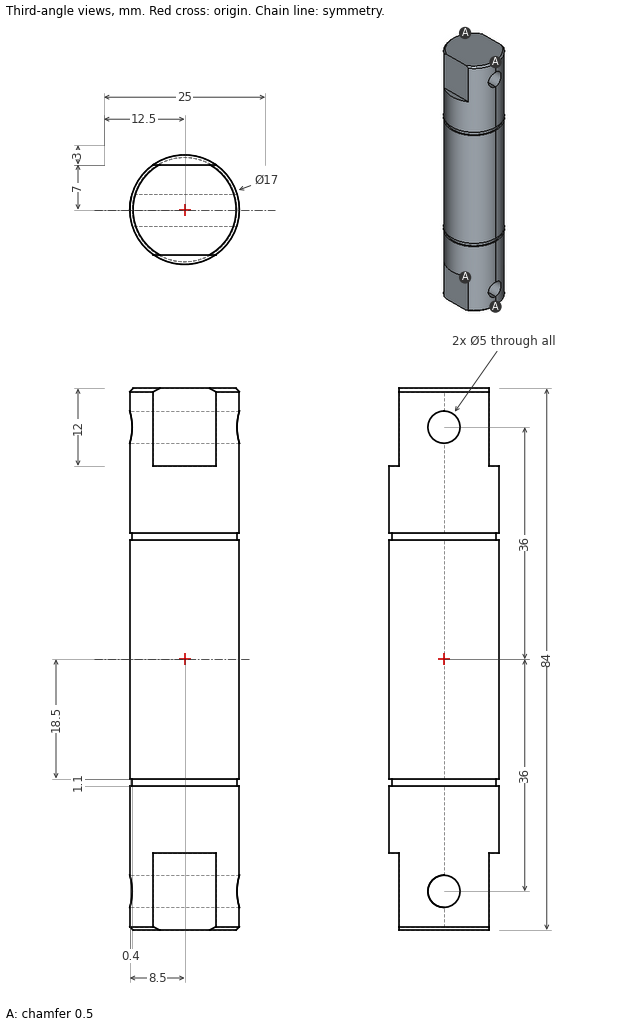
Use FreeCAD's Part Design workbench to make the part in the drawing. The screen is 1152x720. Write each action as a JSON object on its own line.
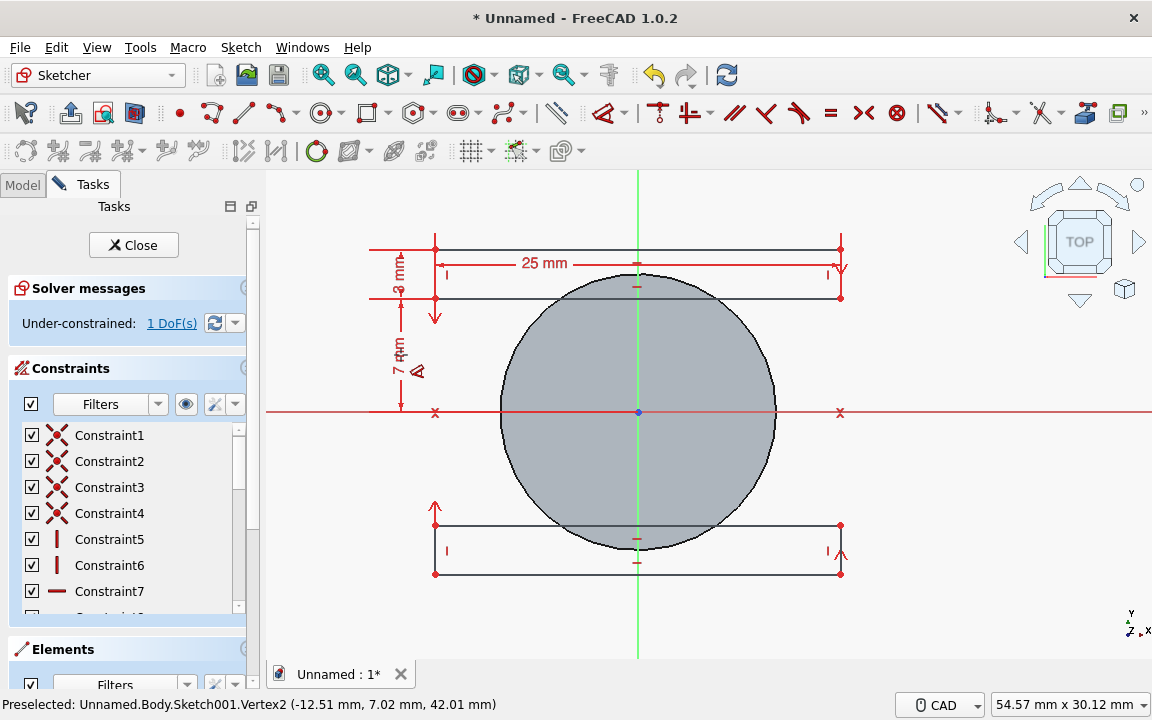
{"action": "left_click", "coordinate": [435, 250]}
{"action": "left_click", "coordinate": [537, 216]}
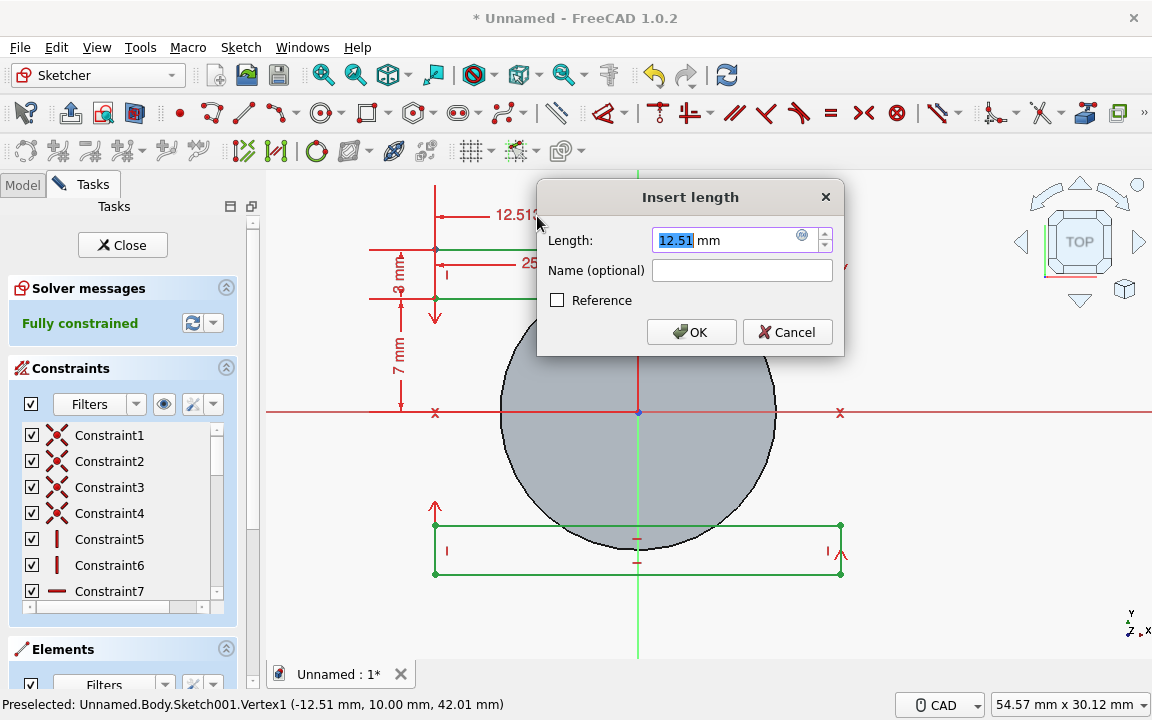
{"action": "type", "text": "12.5"}
{"action": "key", "text": "Return"}
{"action": "key", "text": "Escape"}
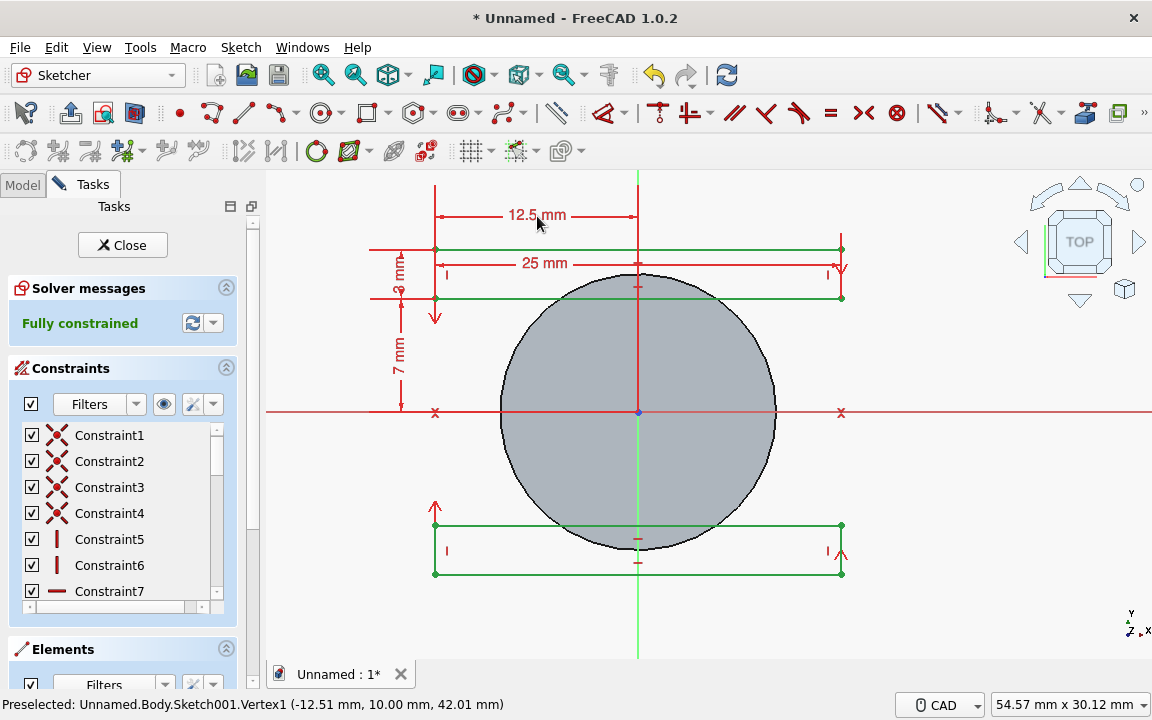
{"action": "left_click", "coordinate": [123, 245]}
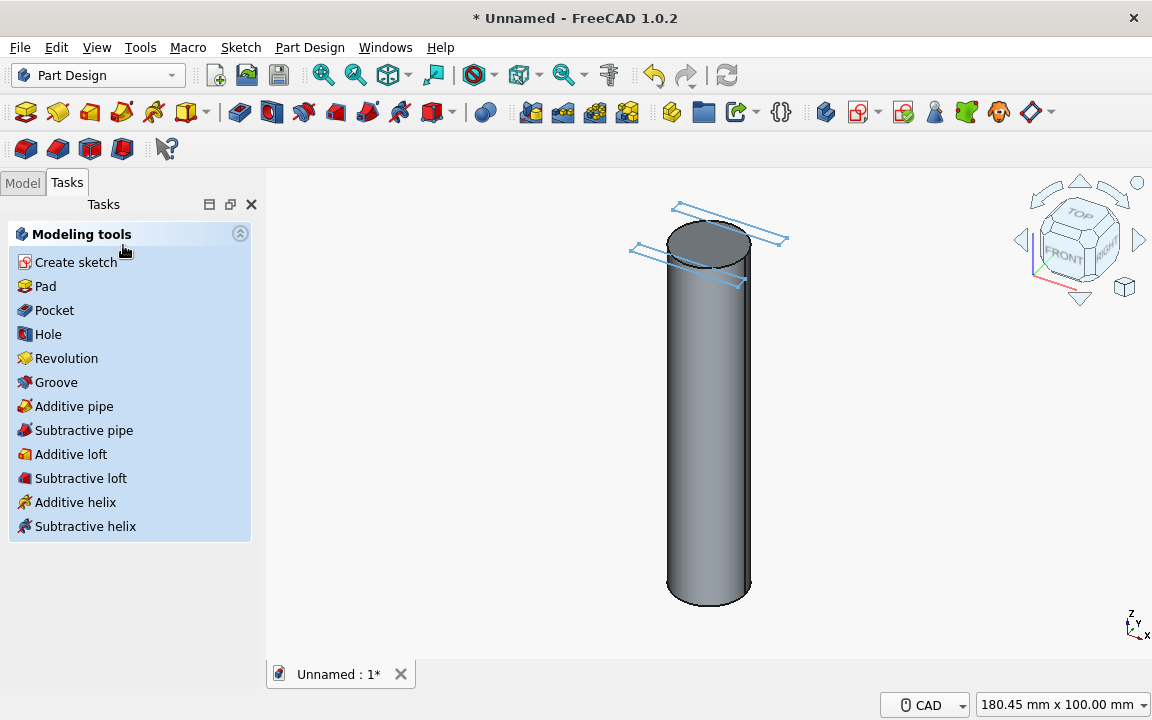
{"action": "left_click", "coordinate": [240, 112]}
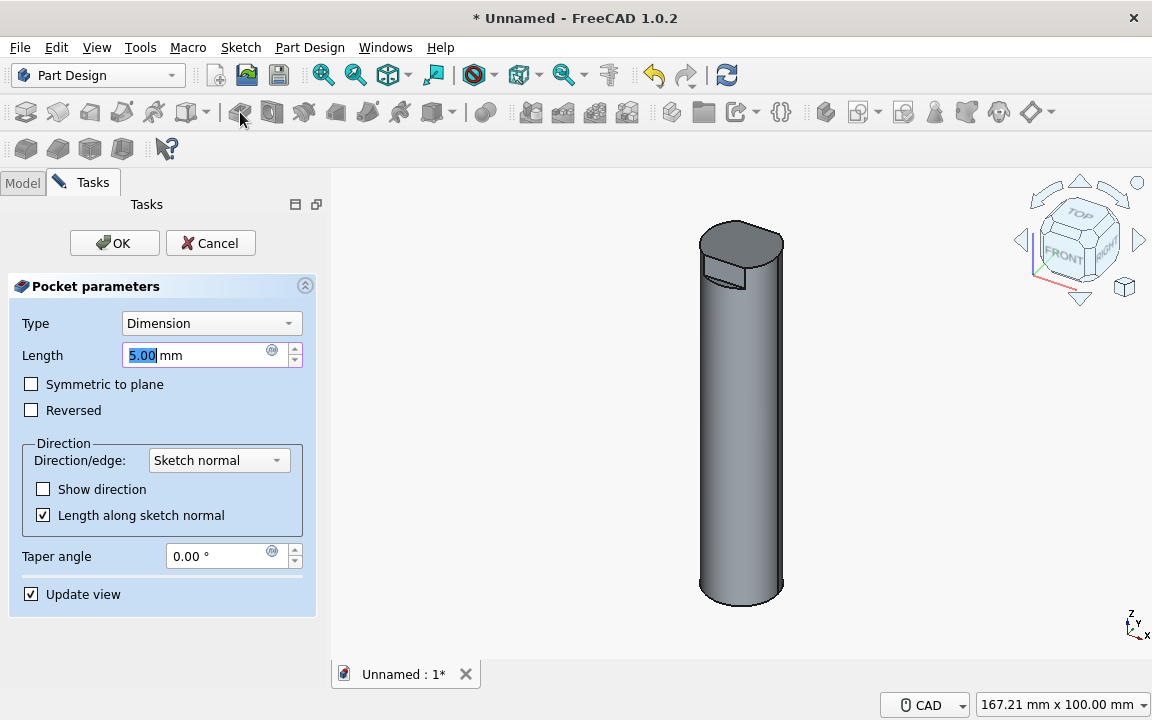
{"action": "type", "text": "12"}
{"action": "key", "text": "Tab"}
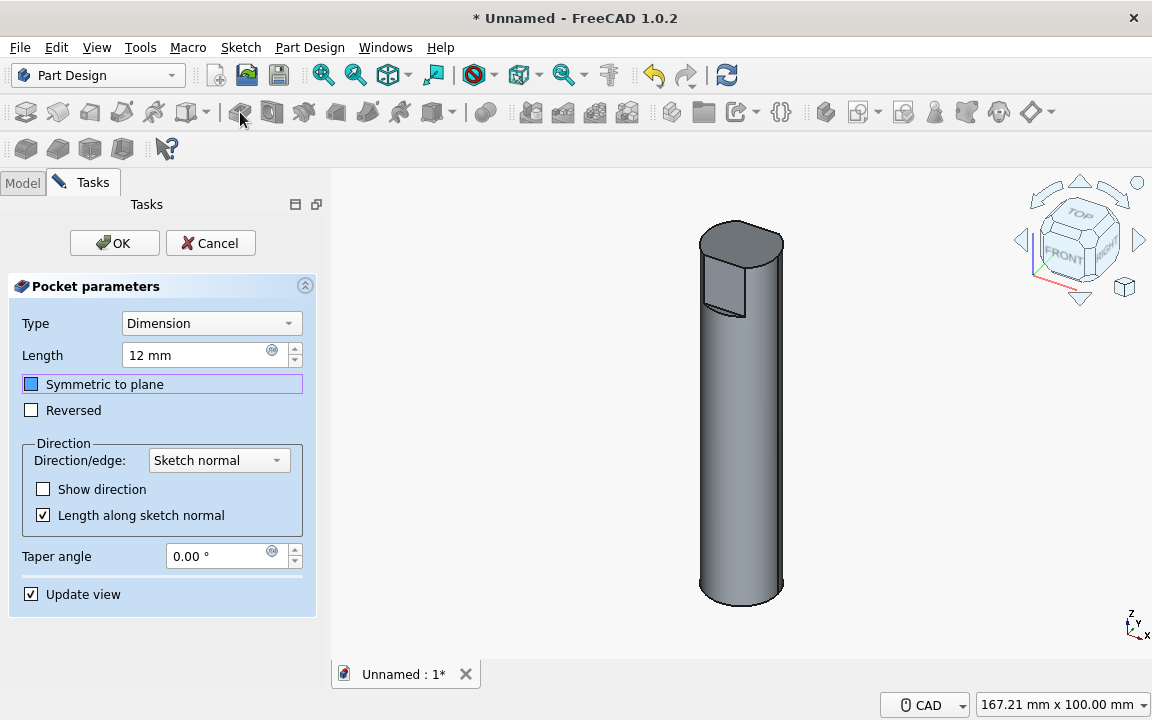
{"action": "left_click", "coordinate": [115, 243]}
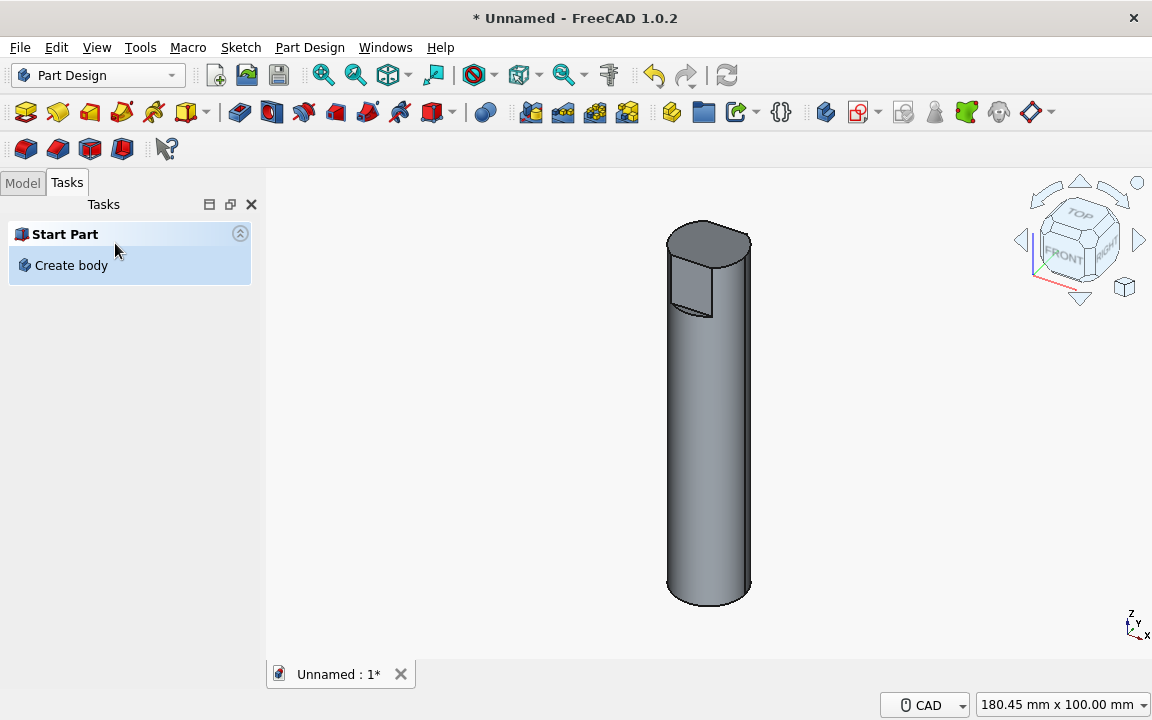
{"action": "left_click", "coordinate": [23, 182]}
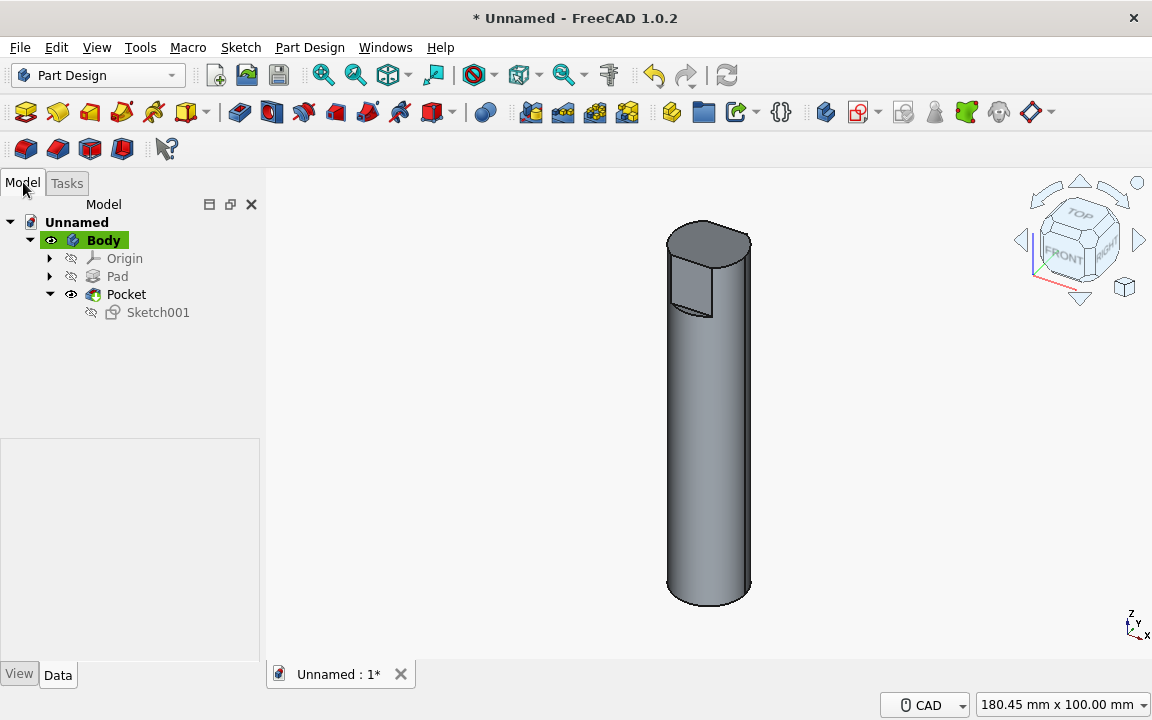
{"action": "left_click", "coordinate": [116, 294]}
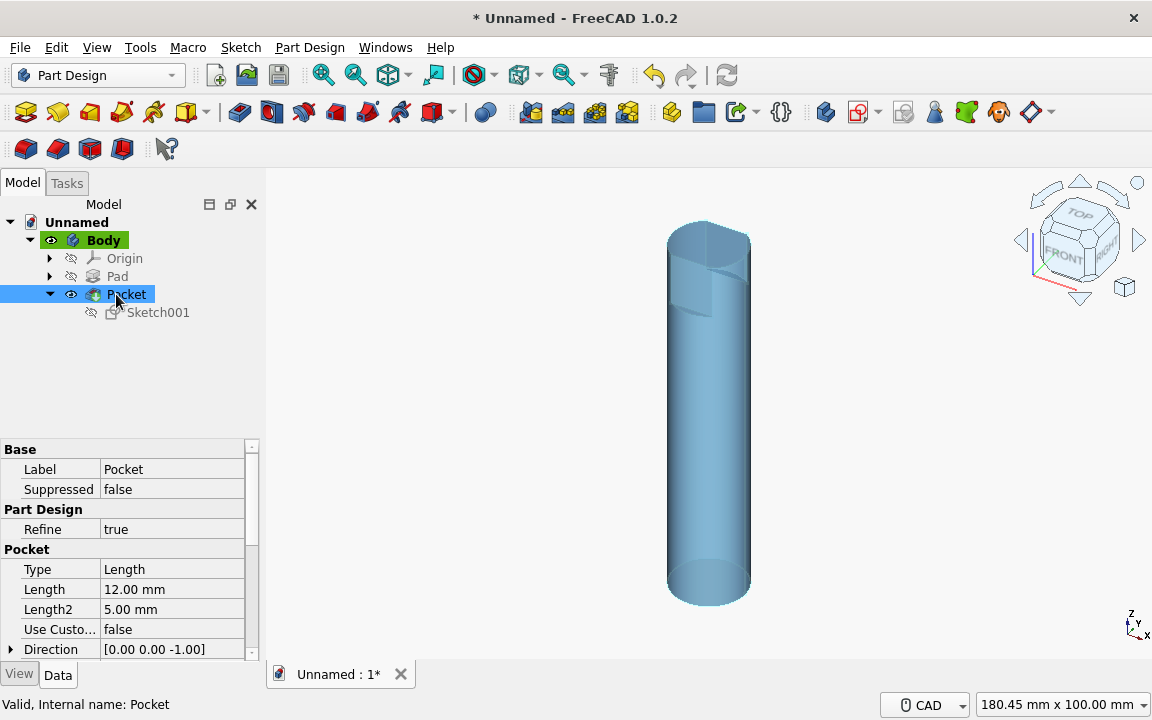
{"action": "left_click", "coordinate": [532, 112]}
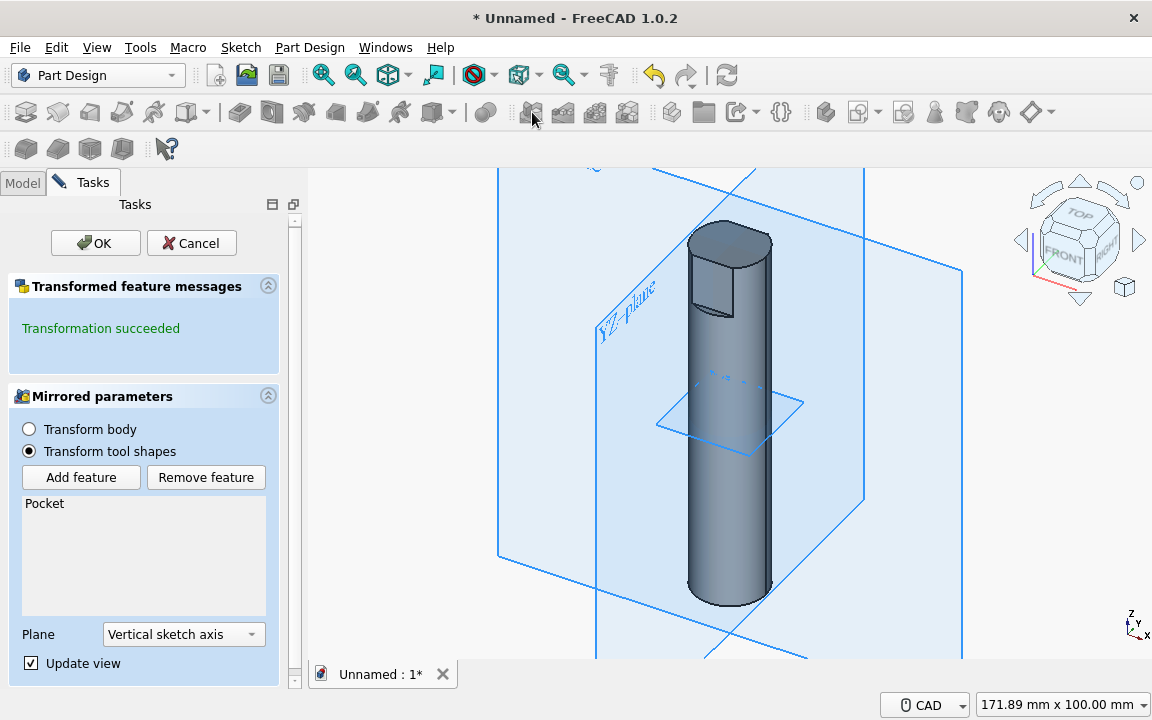
{"action": "left_click", "coordinate": [184, 634]}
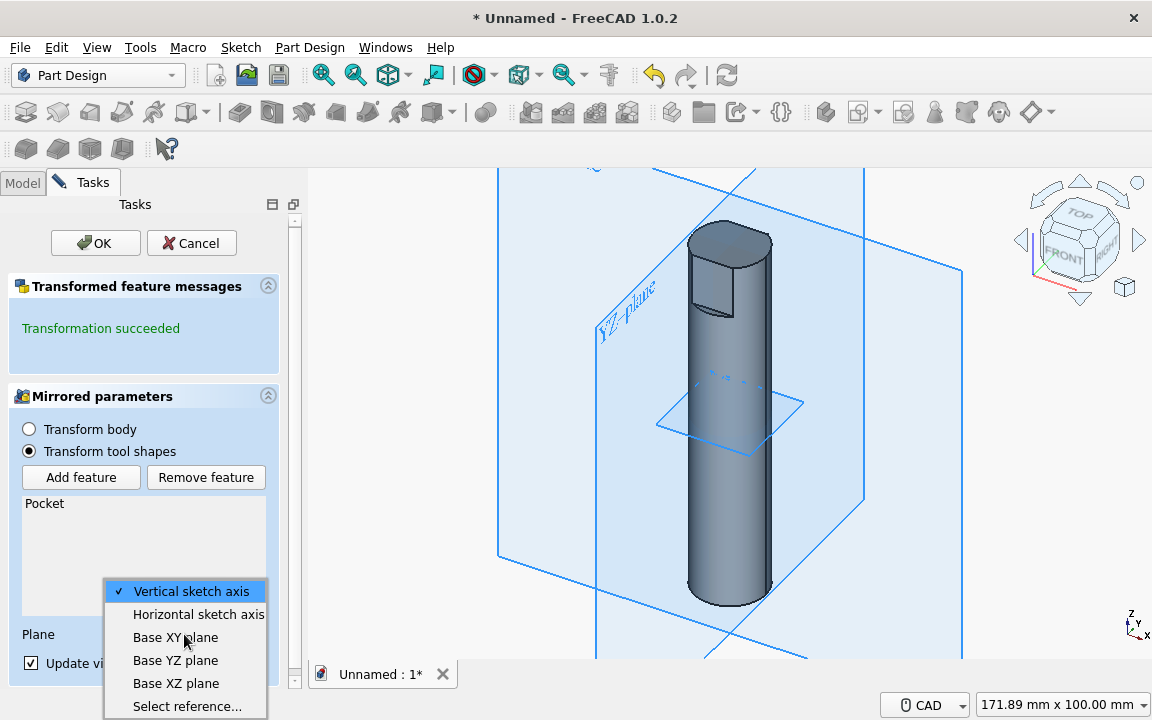
{"action": "left_click", "coordinate": [184, 638]}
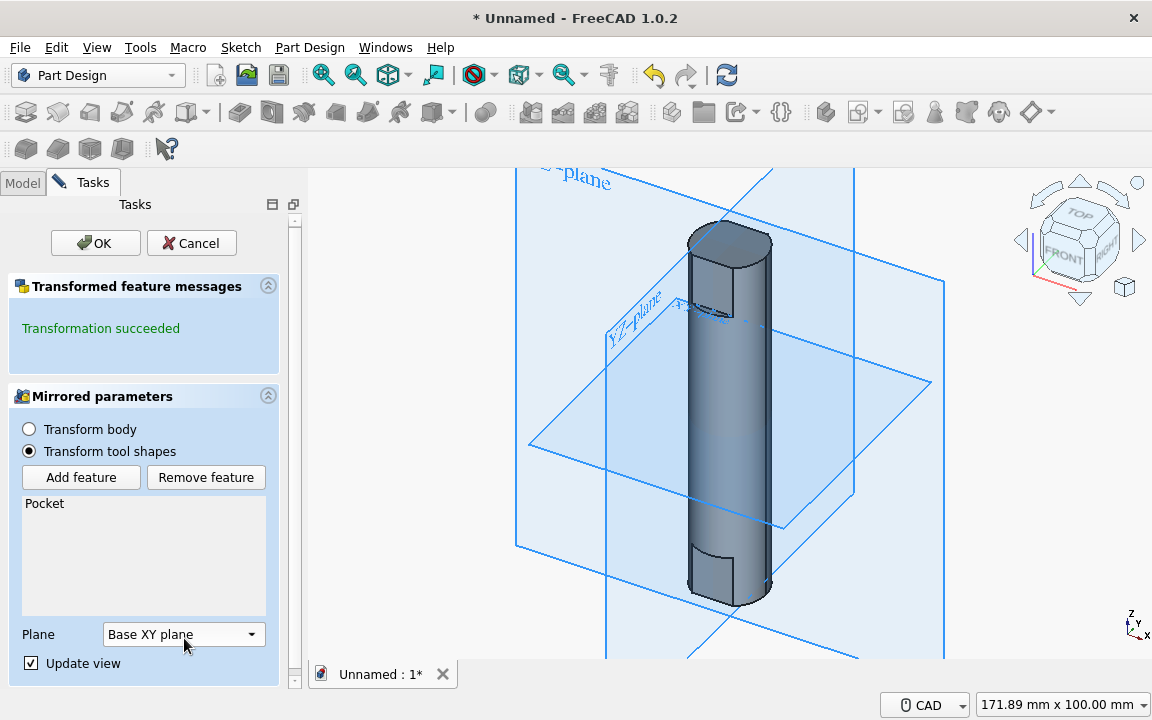
{"action": "left_click", "coordinate": [96, 243]}